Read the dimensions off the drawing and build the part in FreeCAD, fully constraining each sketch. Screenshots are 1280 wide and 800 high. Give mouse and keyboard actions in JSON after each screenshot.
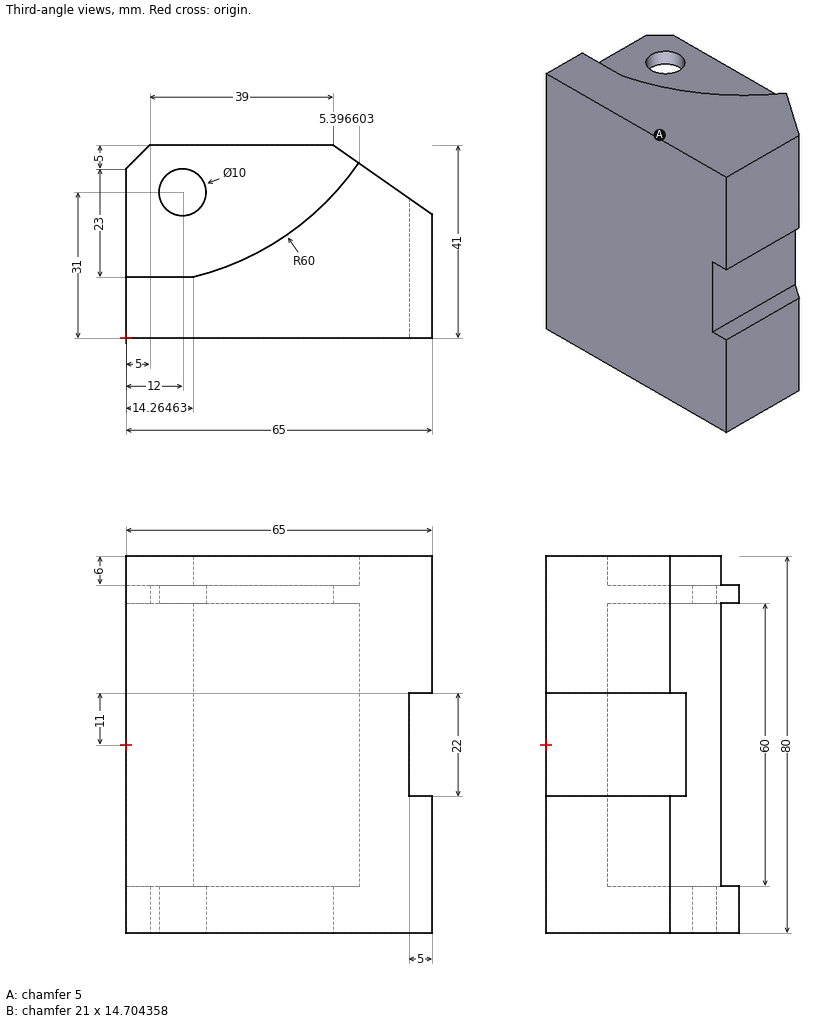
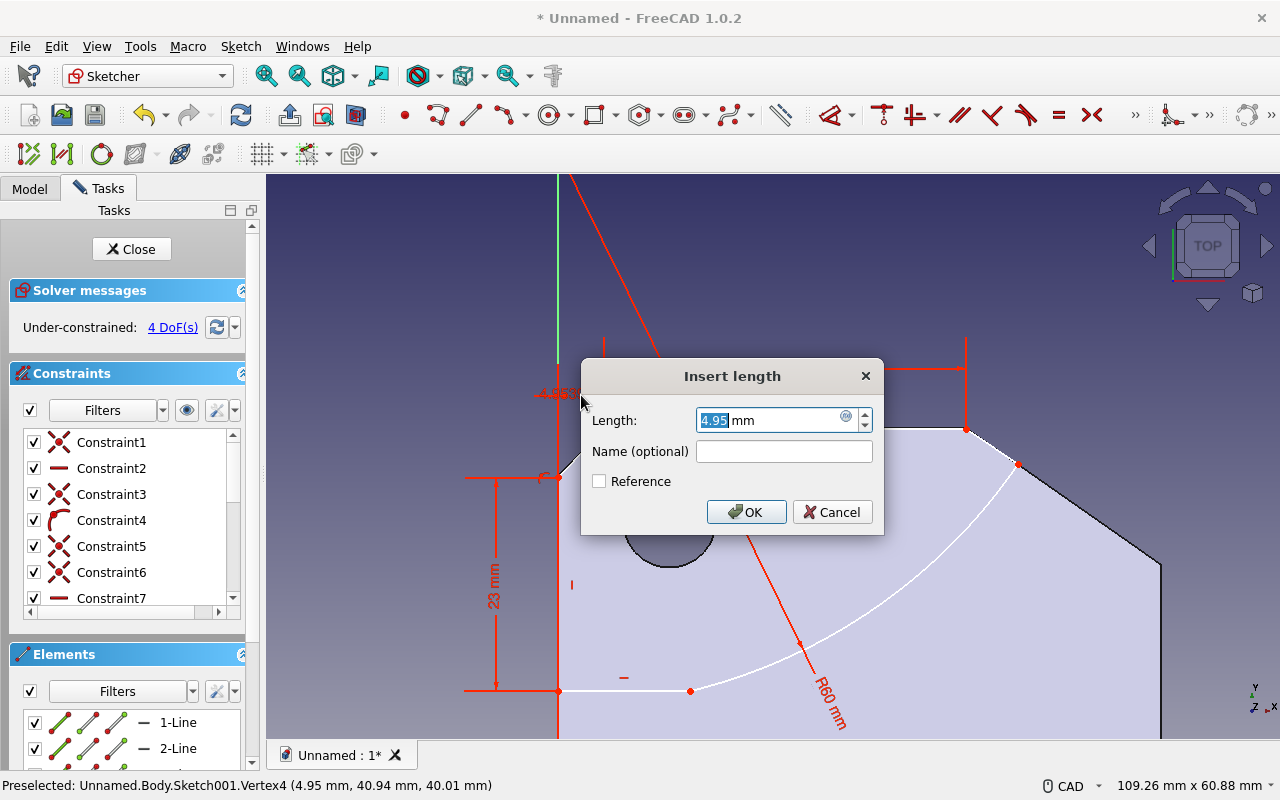
{"action": "type", "text": "5"}
{"action": "key", "text": "Return"}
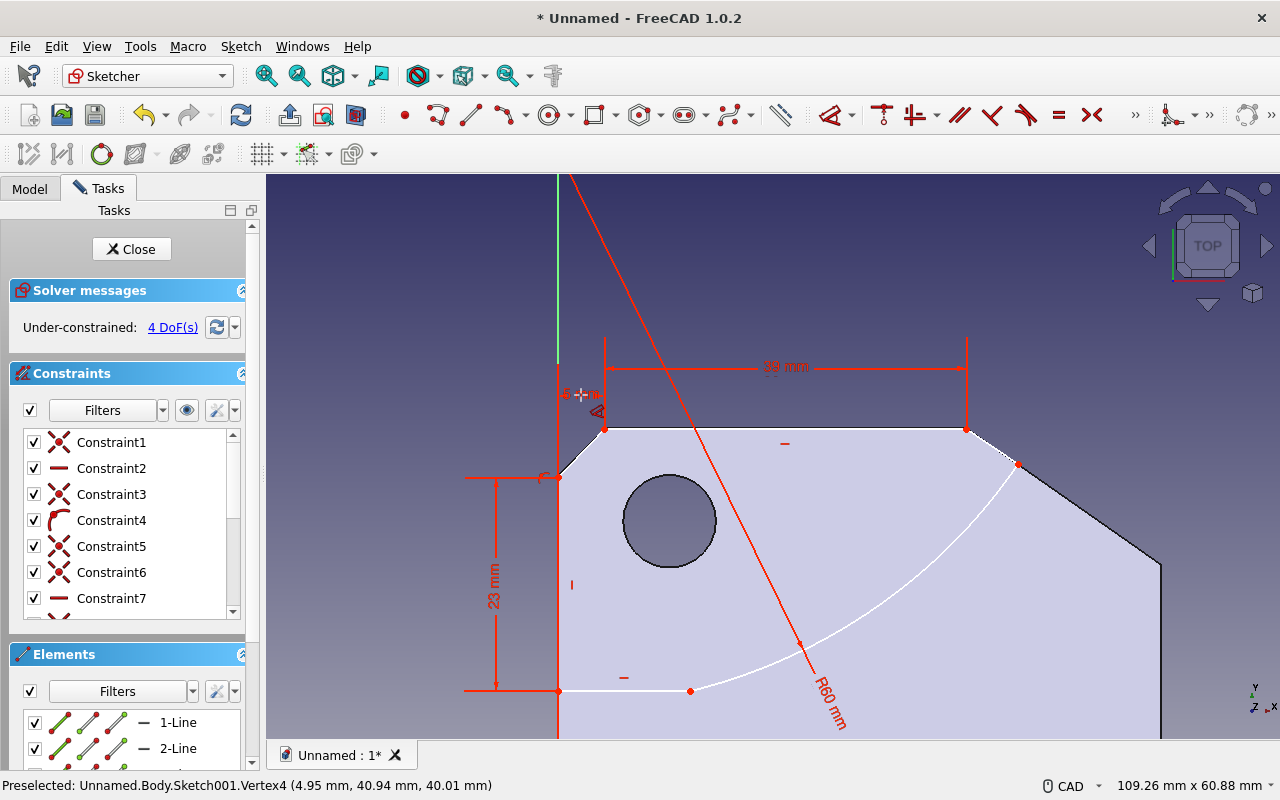
{"action": "left_click", "coordinate": [591, 444]}
{"action": "left_click", "coordinate": [524, 453]}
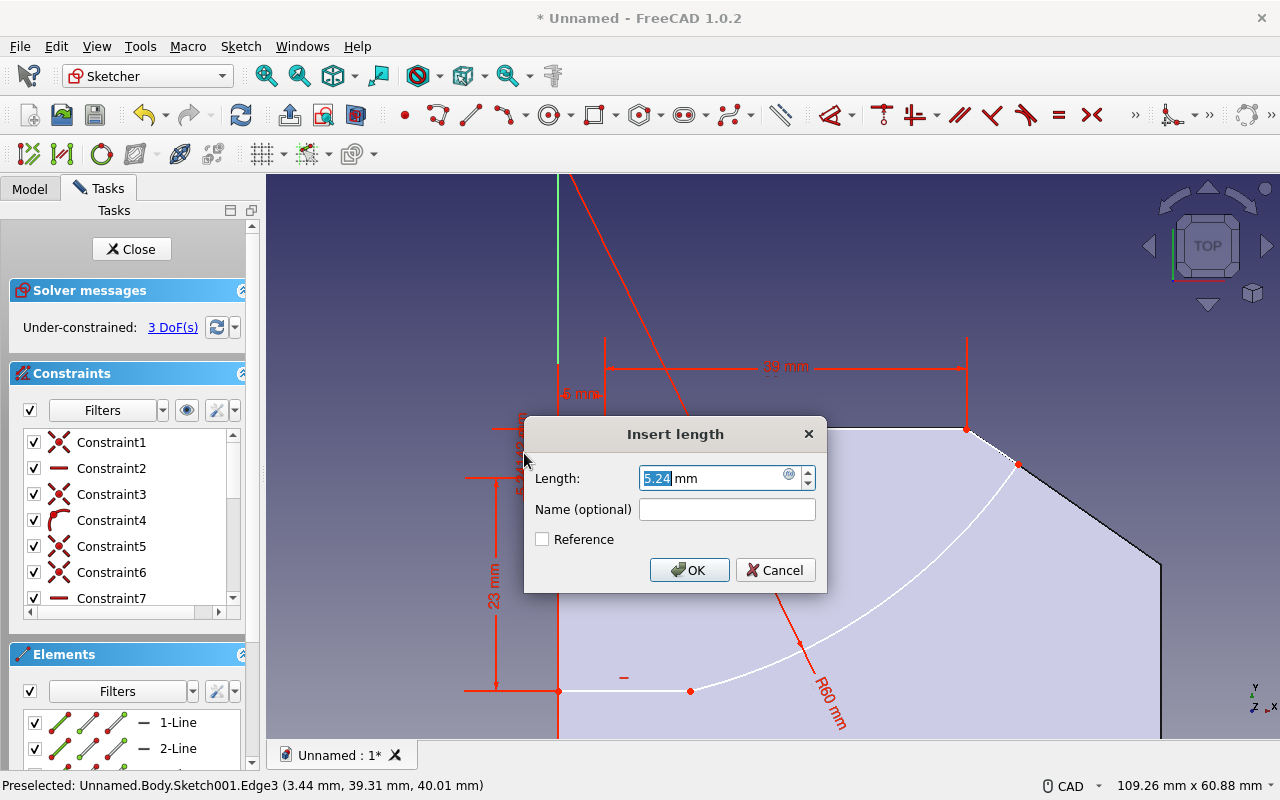
{"action": "type", "text": "5"}
{"action": "key", "text": "Return"}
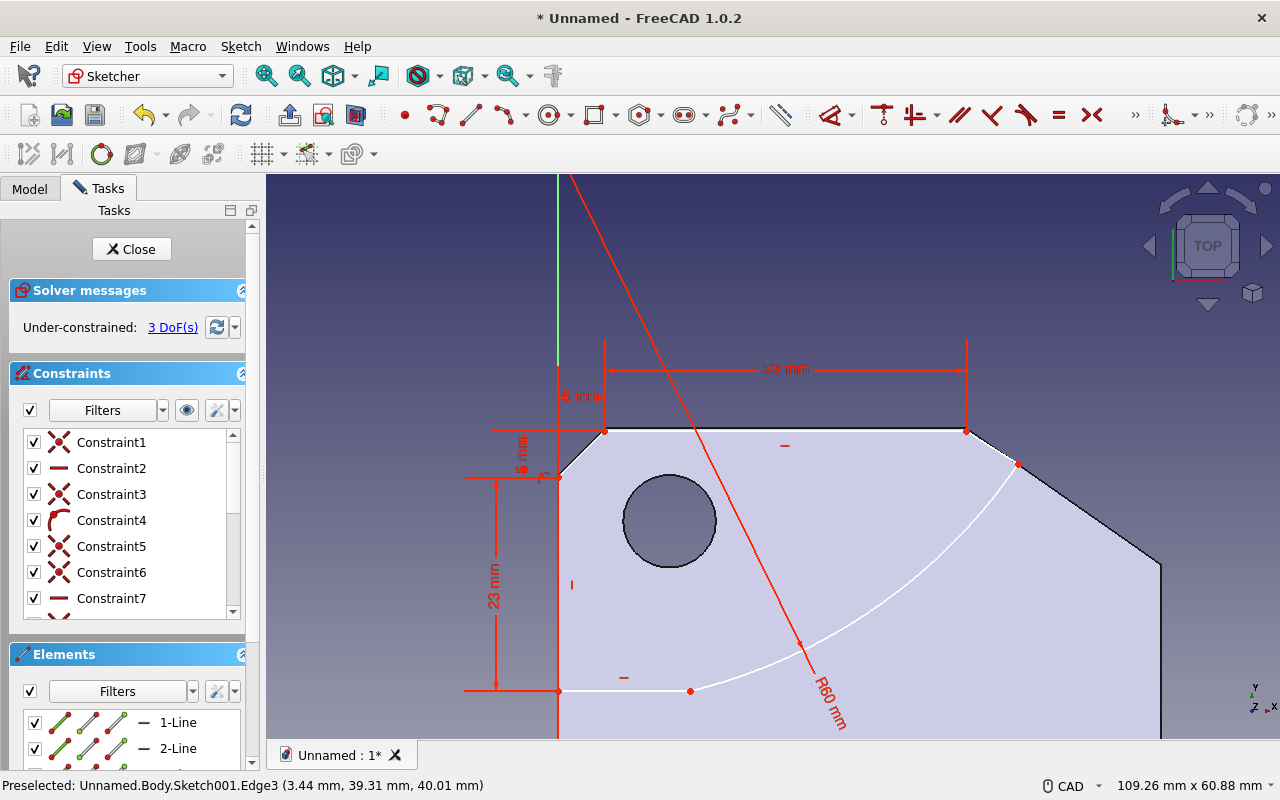
{"action": "left_click", "coordinate": [967, 431]}
{"action": "left_click", "coordinate": [524, 507]}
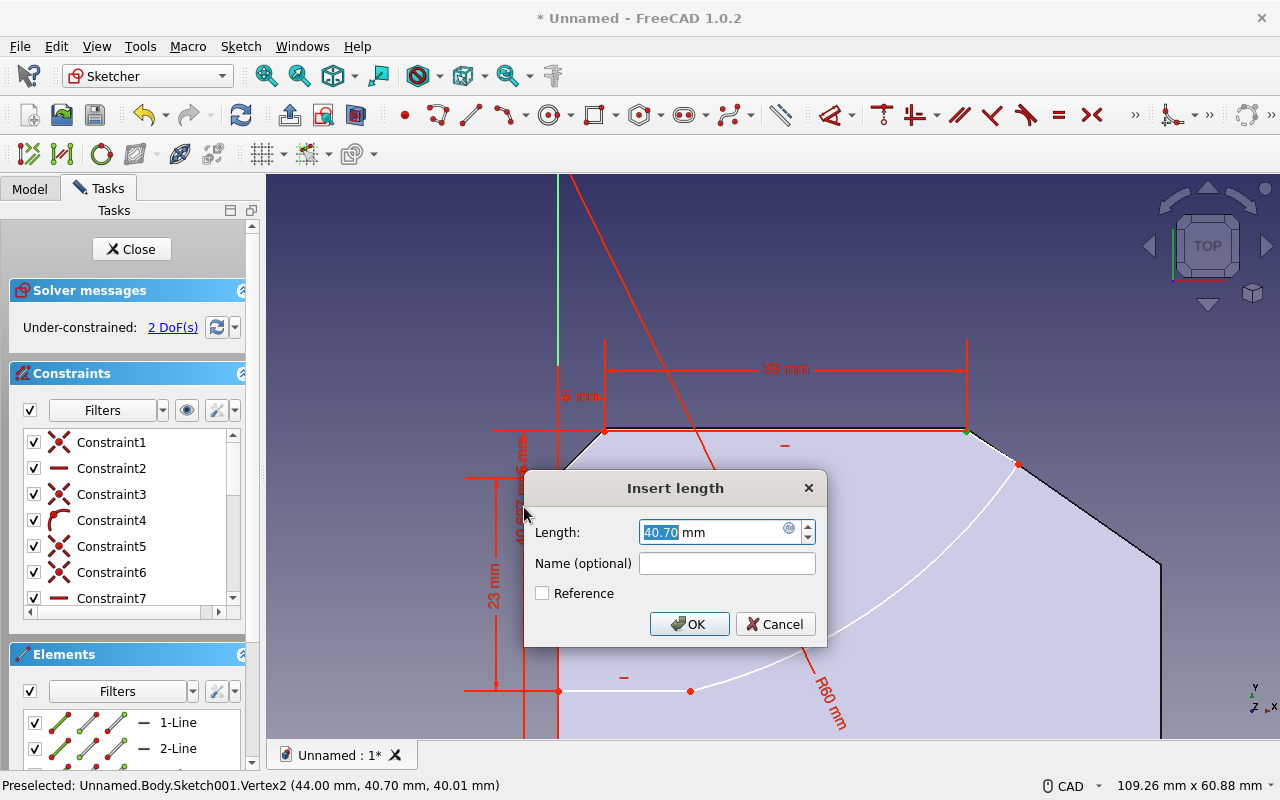
{"action": "type", "text": "41"}
{"action": "key", "text": "Return"}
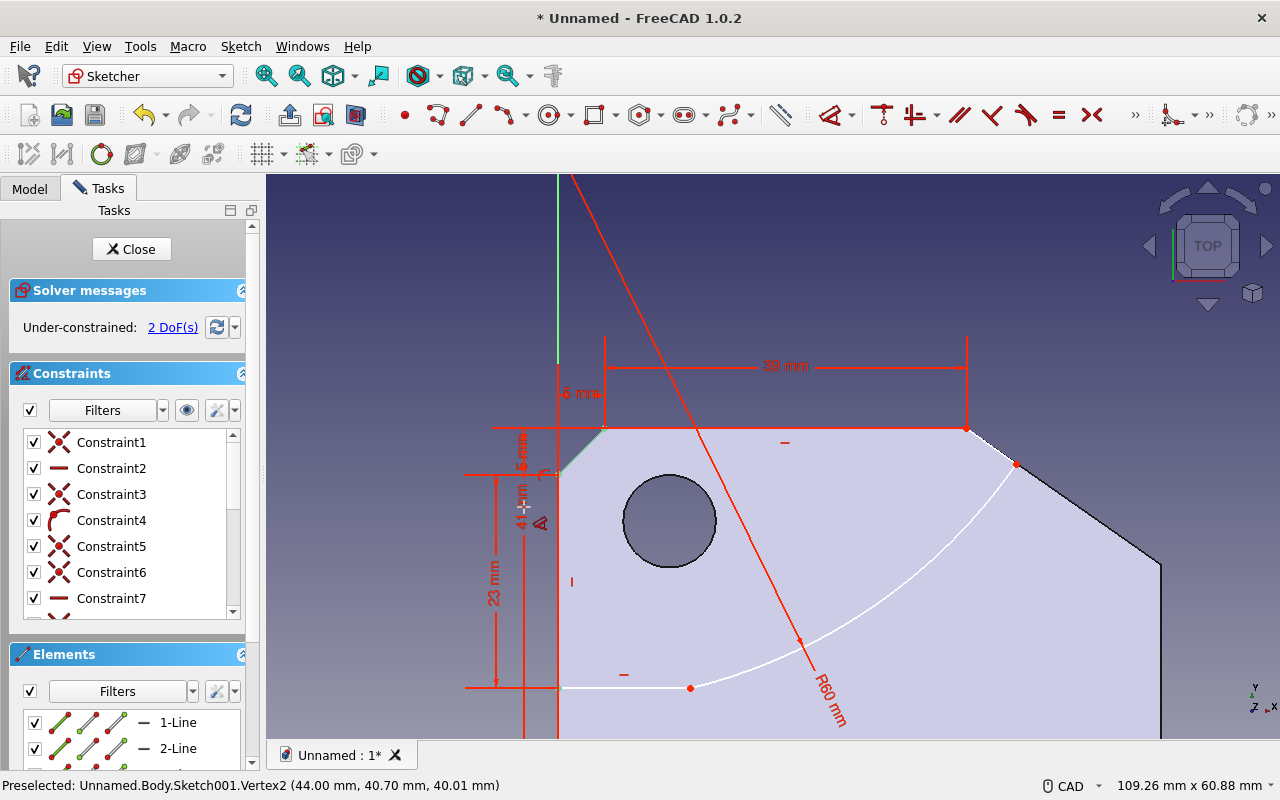
{"action": "left_click", "coordinate": [598, 688]}
{"action": "left_click", "coordinate": [624, 654]}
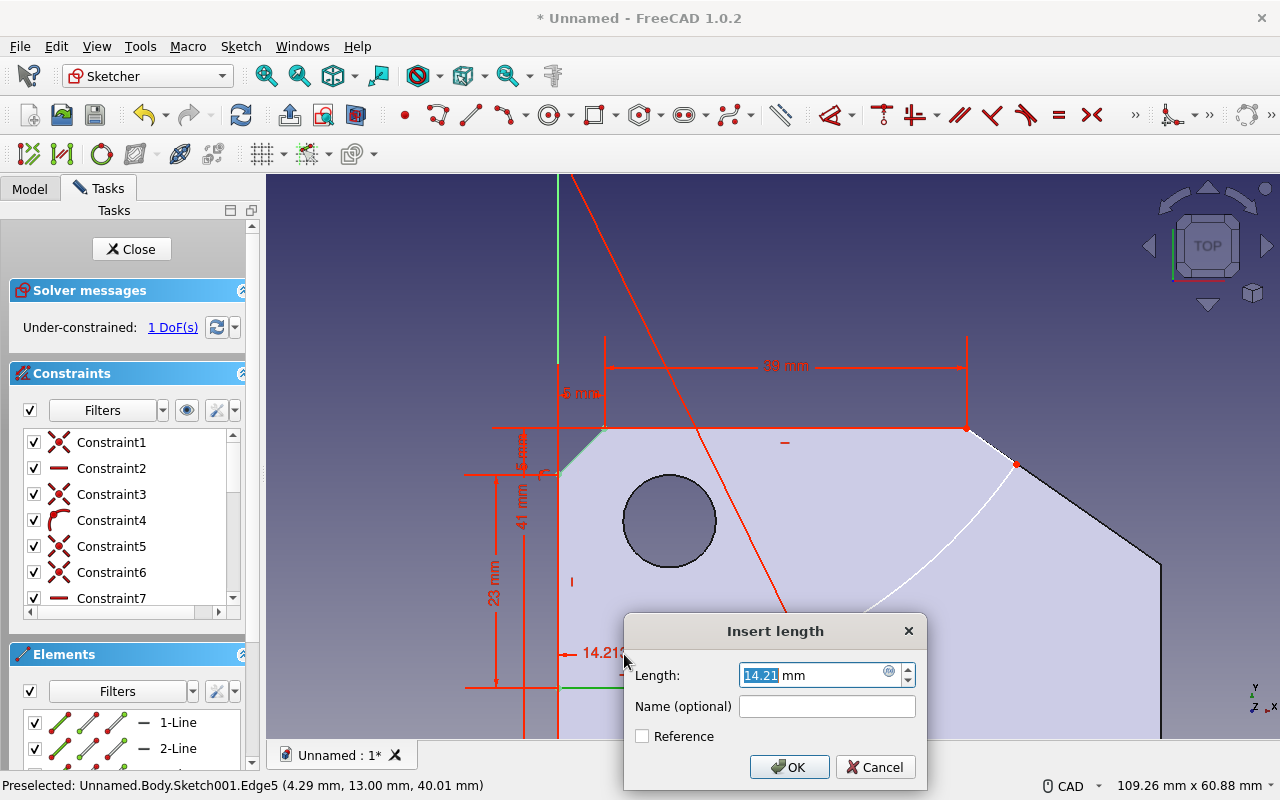
{"action": "type", "text": "14.26463"}
{"action": "key", "text": "Return"}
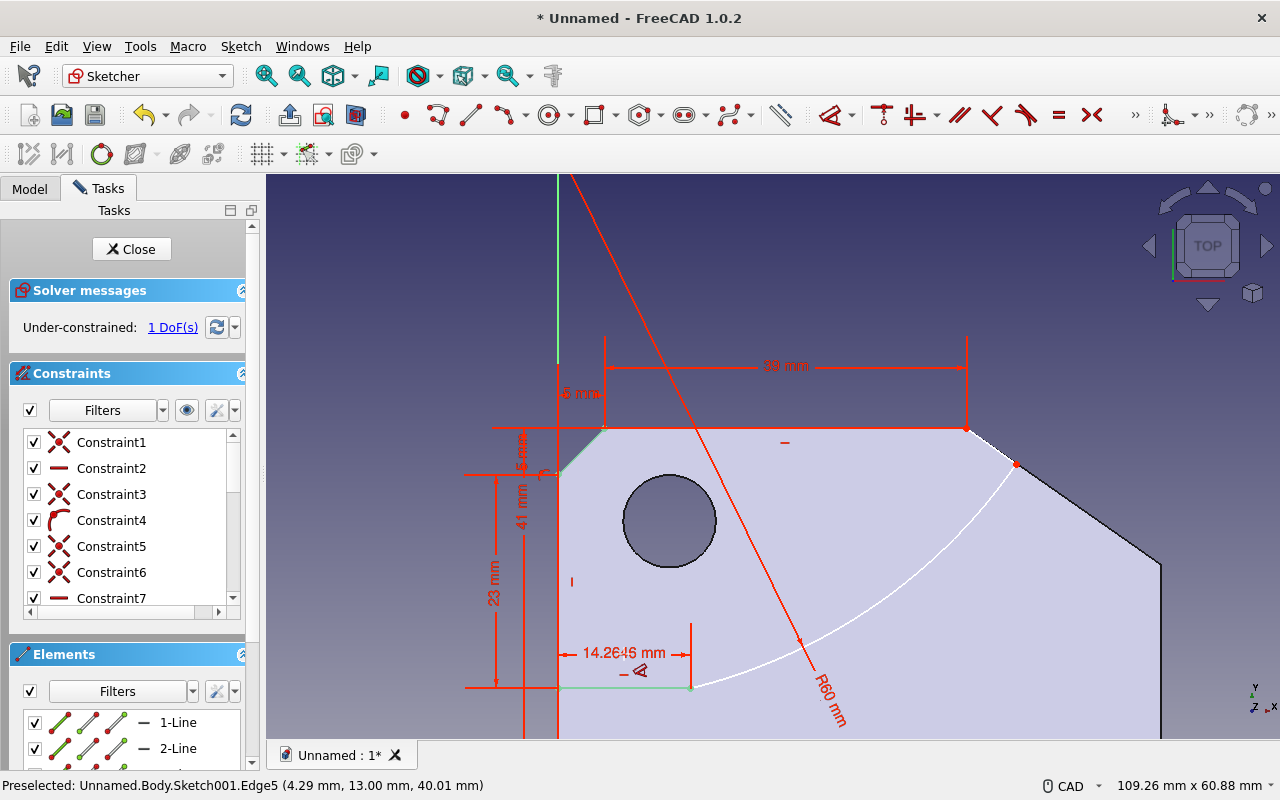
{"action": "left_click", "coordinate": [1001, 453]}
{"action": "left_click", "coordinate": [991, 394]}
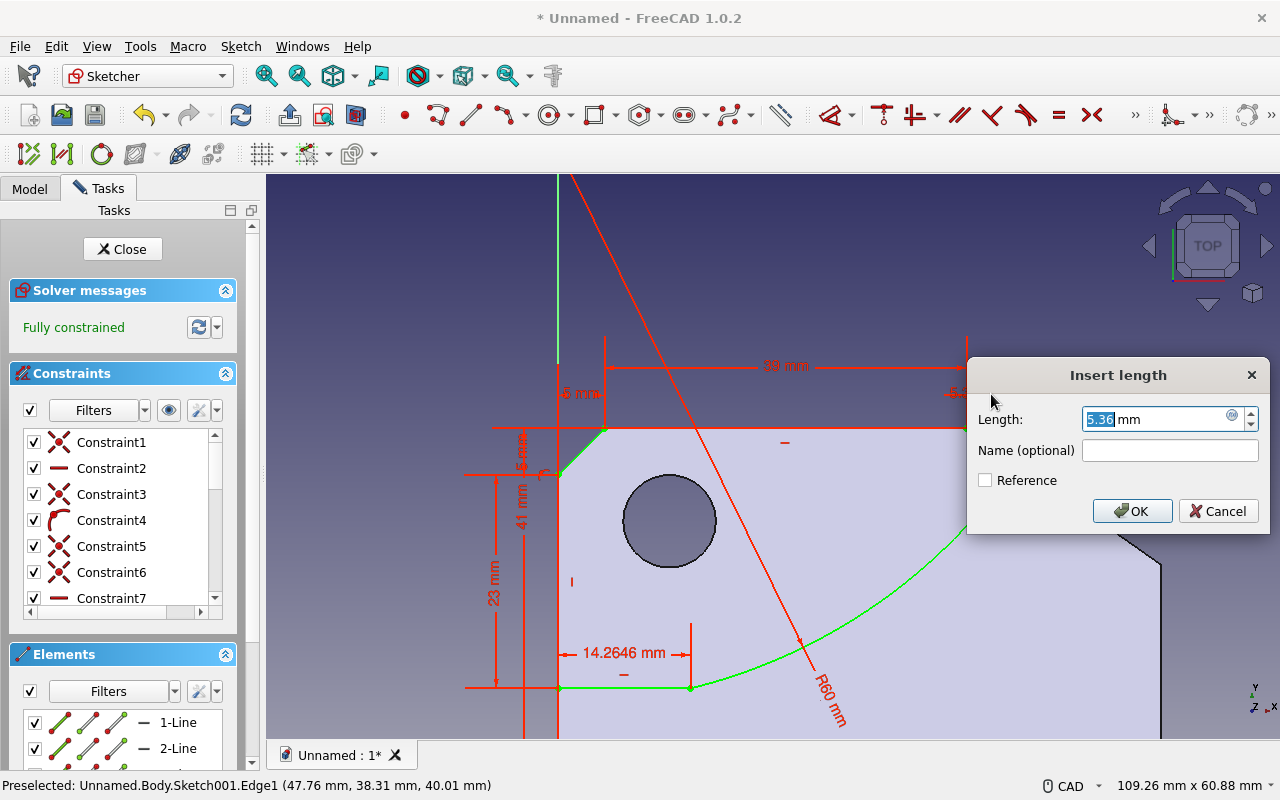
{"action": "type", "text": "5.396603"}
{"action": "key", "text": "Return"}
{"action": "key", "text": "Escape"}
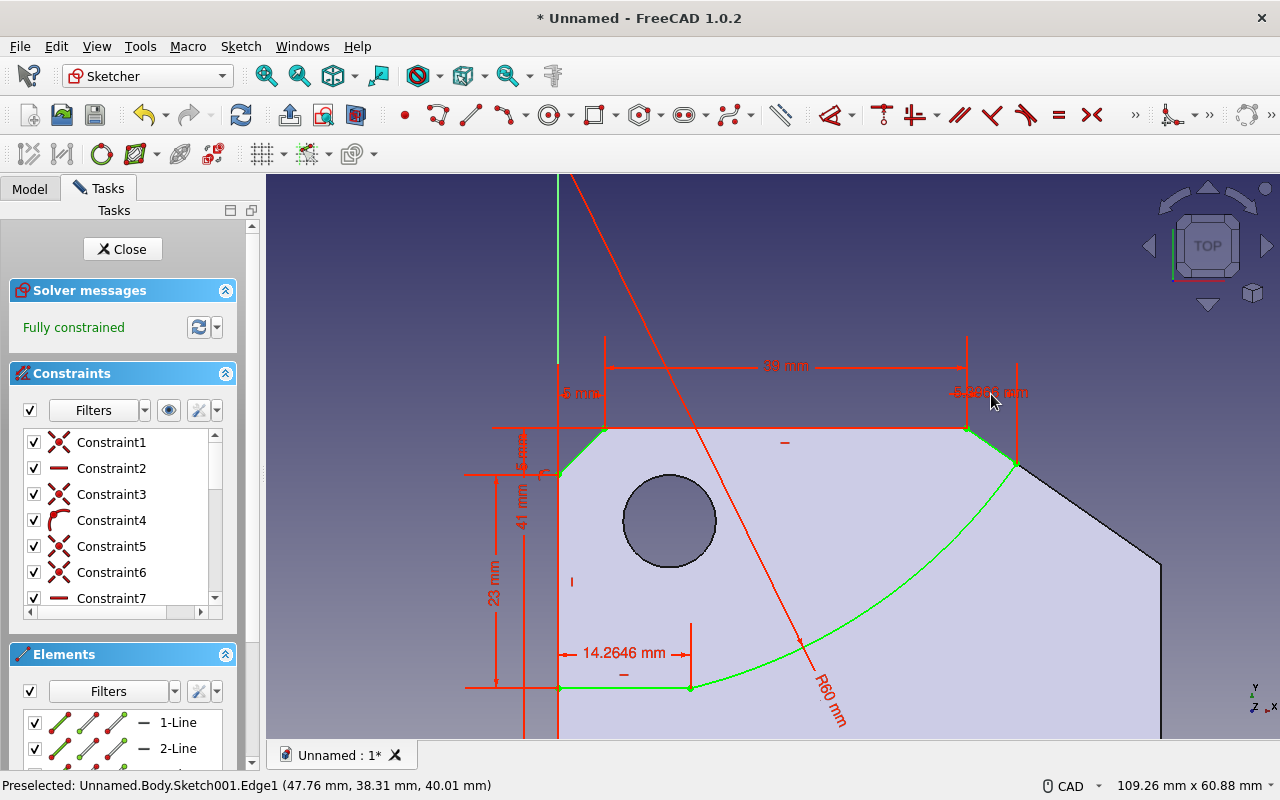
{"action": "left_click", "coordinate": [123, 249]}